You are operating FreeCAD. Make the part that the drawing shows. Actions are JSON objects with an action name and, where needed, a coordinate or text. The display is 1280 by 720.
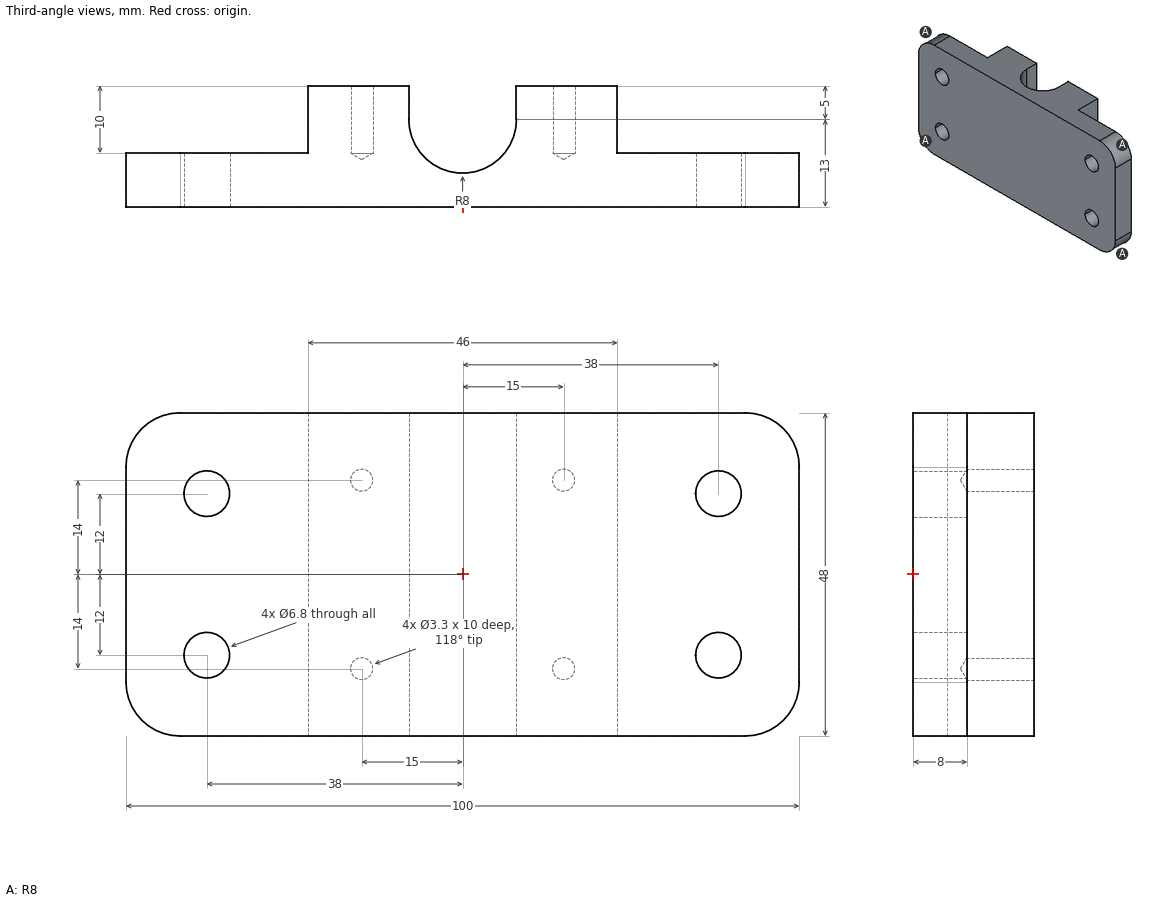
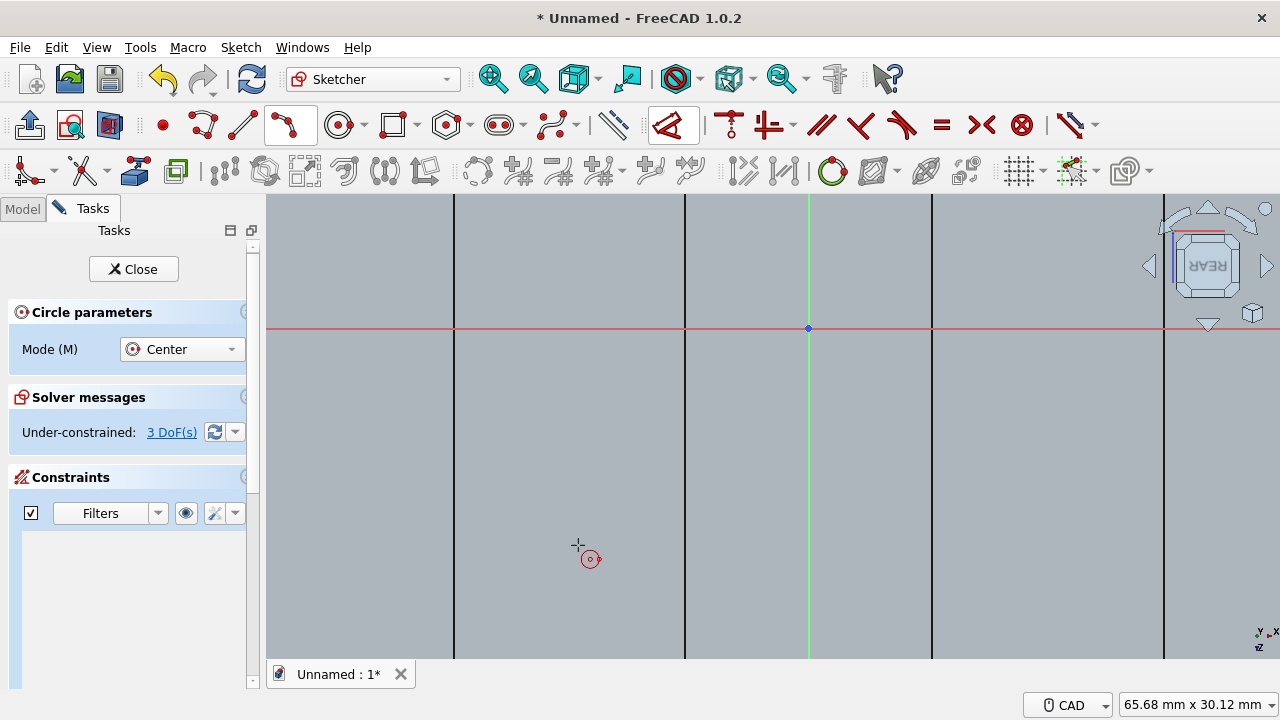
{"action": "left_click", "coordinate": [577, 545]}
{"action": "left_click", "coordinate": [595, 527]}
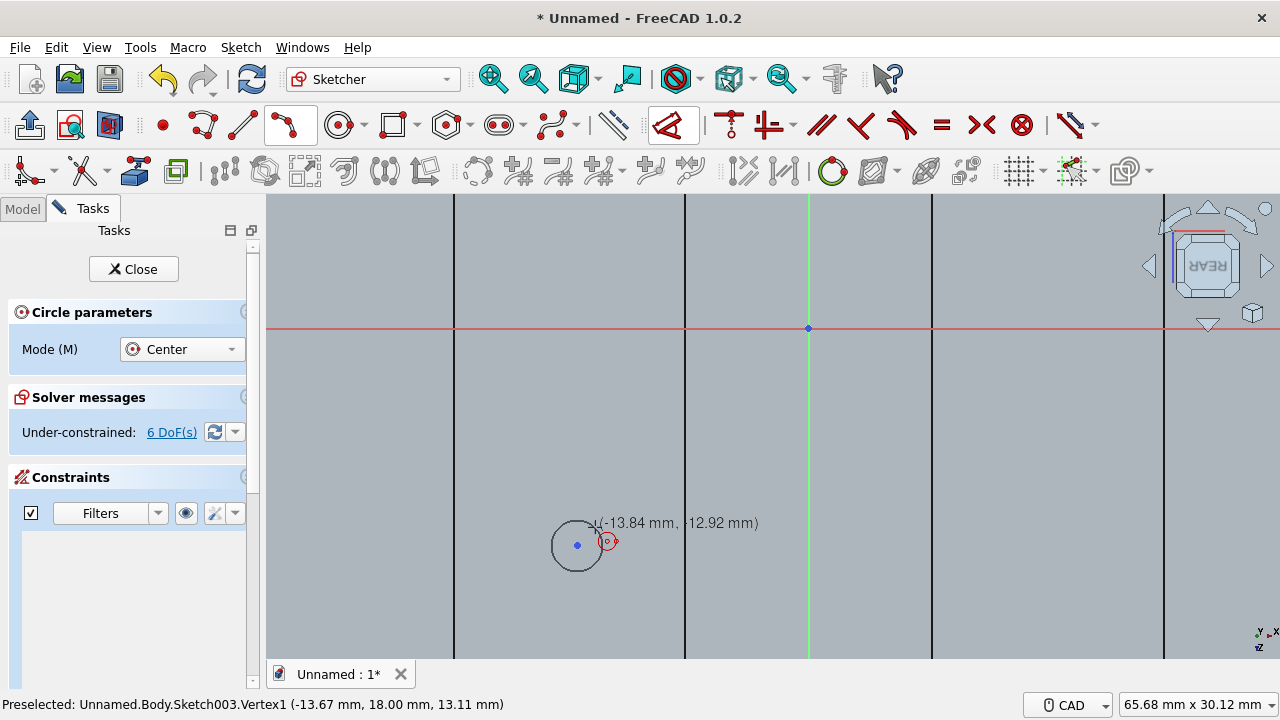
{"action": "left_click", "coordinate": [1040, 545]}
{"action": "left_click", "coordinate": [1058, 527]}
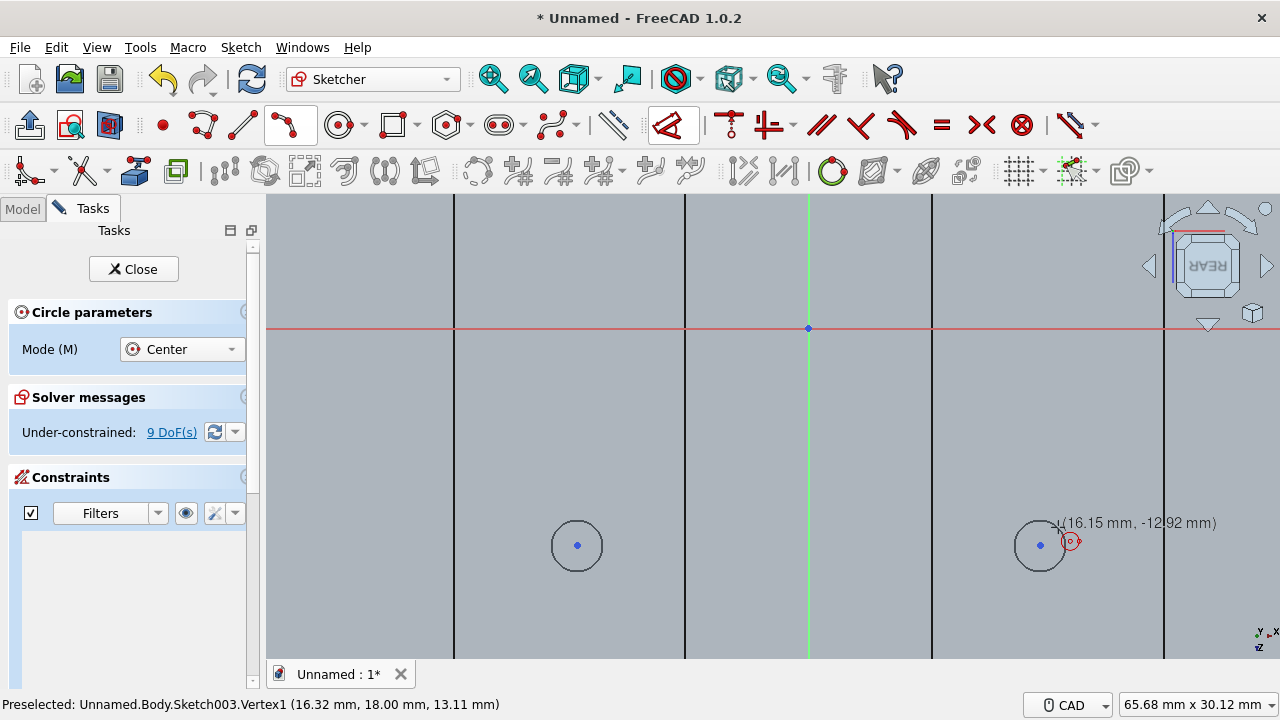
{"action": "scroll", "coordinate": [578, 546], "scroll_direction": "down", "scroll_amount": 3}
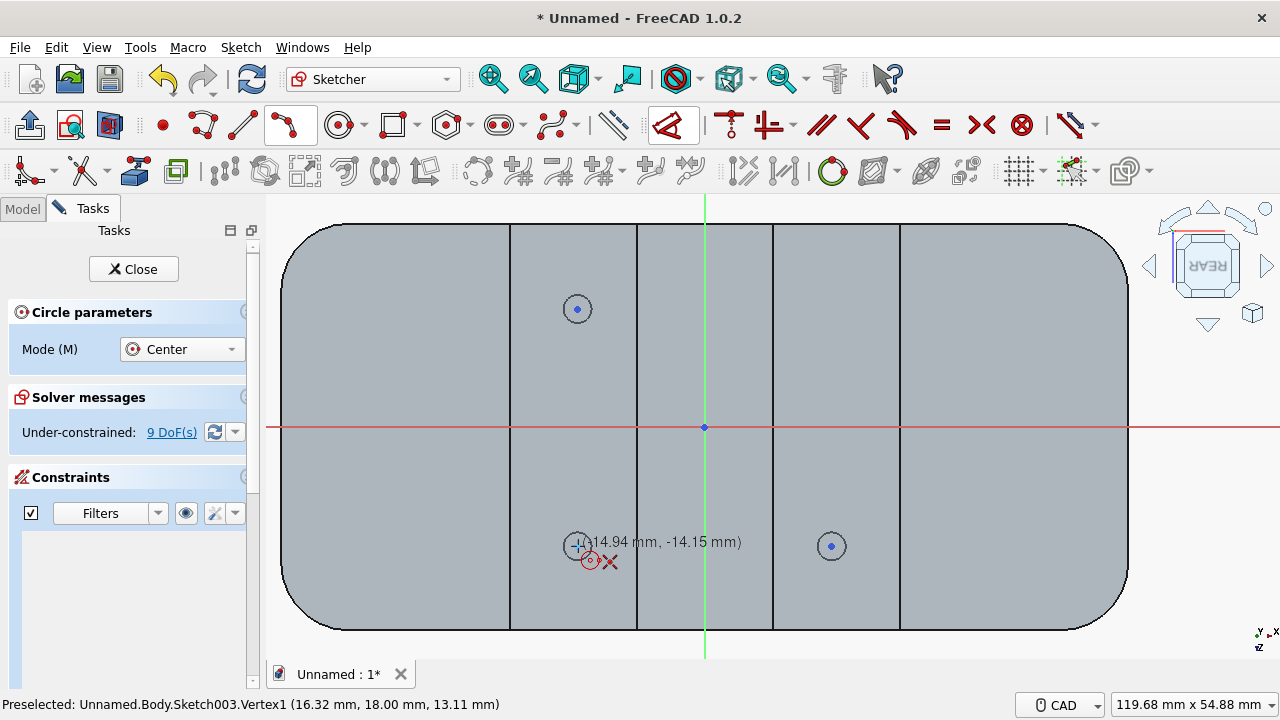
{"action": "scroll", "coordinate": [832, 308], "scroll_direction": "up", "scroll_amount": 3}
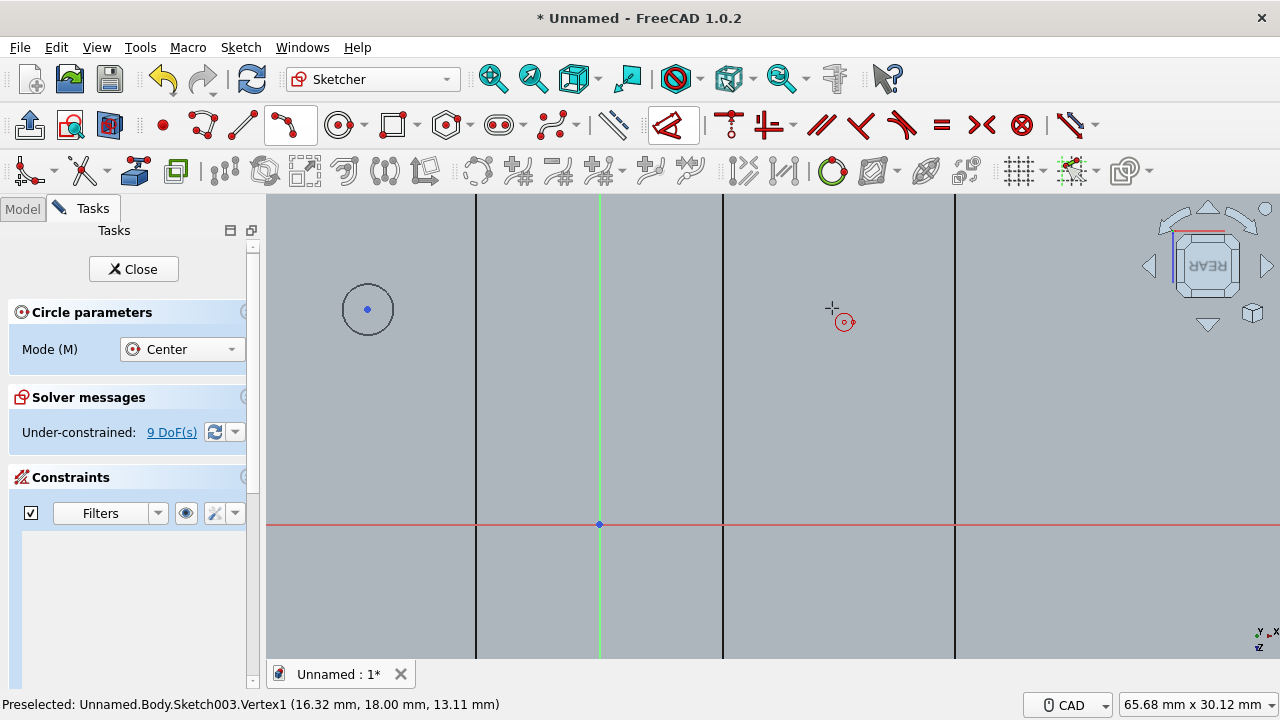
{"action": "left_click", "coordinate": [831, 309]}
{"action": "left_click", "coordinate": [849, 291]}
{"action": "key", "text": "Escape"}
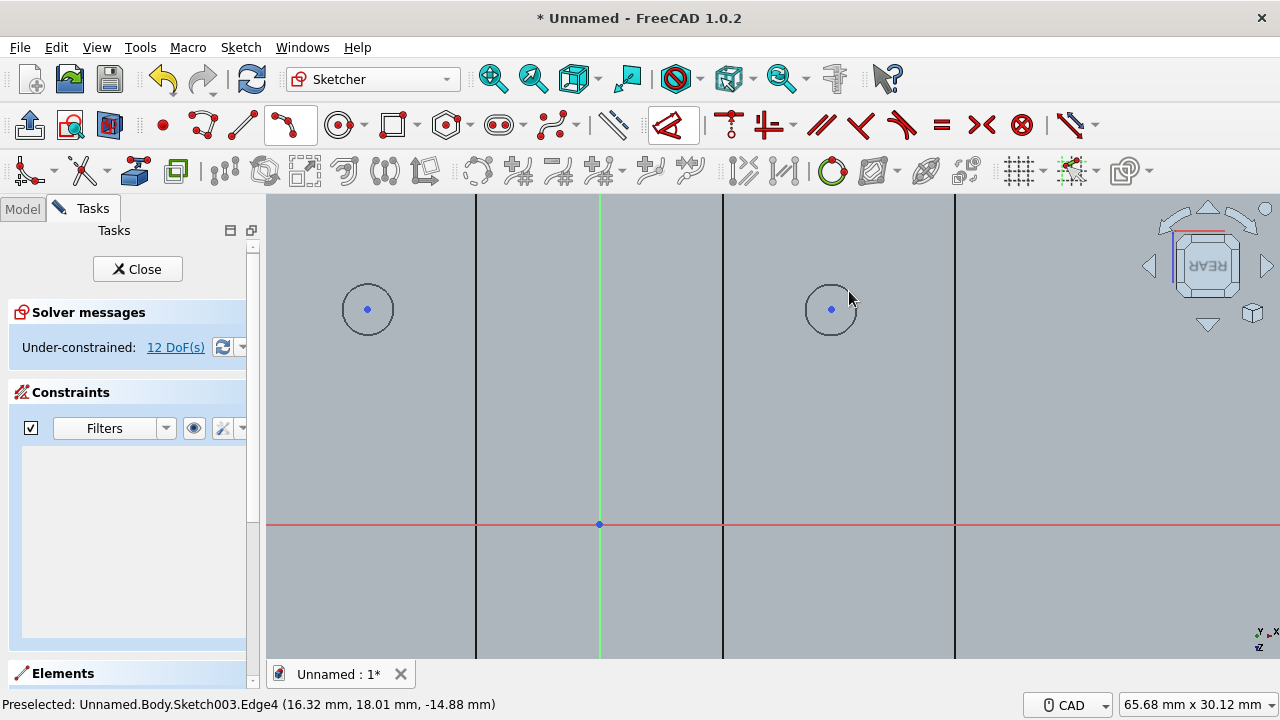
{"action": "left_click", "coordinate": [386, 292]}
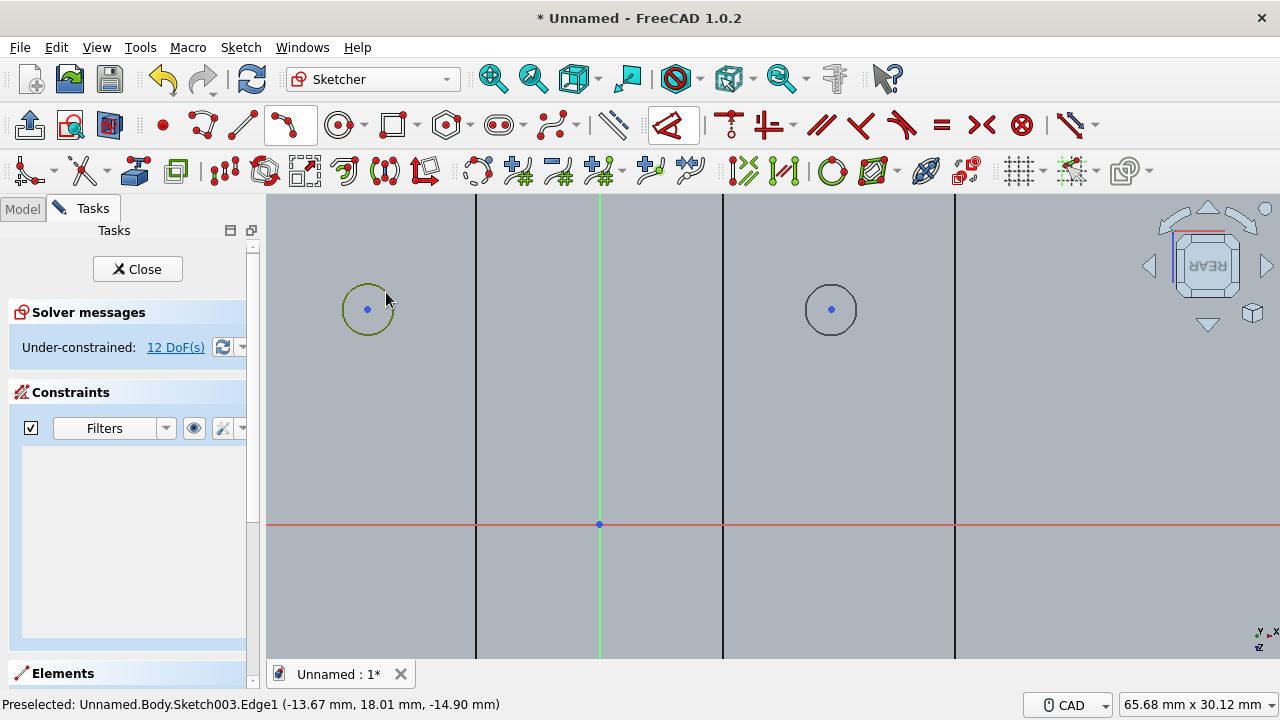
{"action": "scroll", "coordinate": [832, 307], "scroll_direction": "down", "scroll_amount": 3}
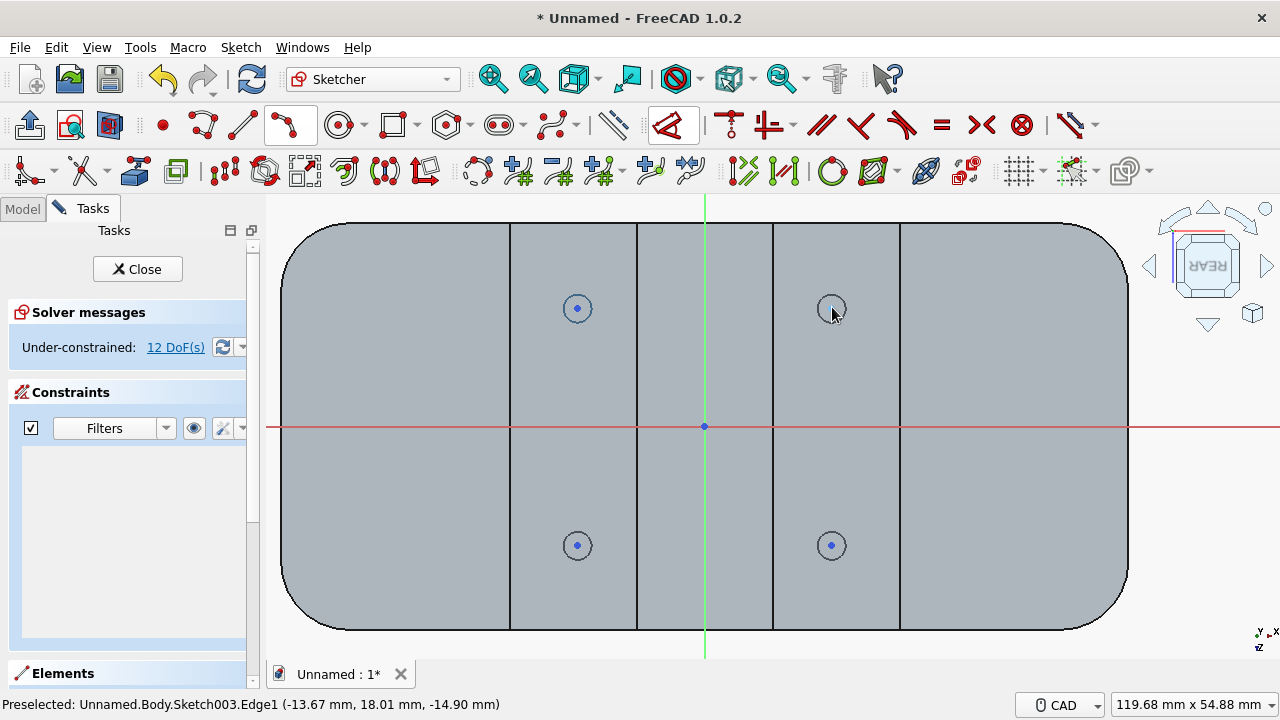
{"action": "left_click", "coordinate": [587, 536]}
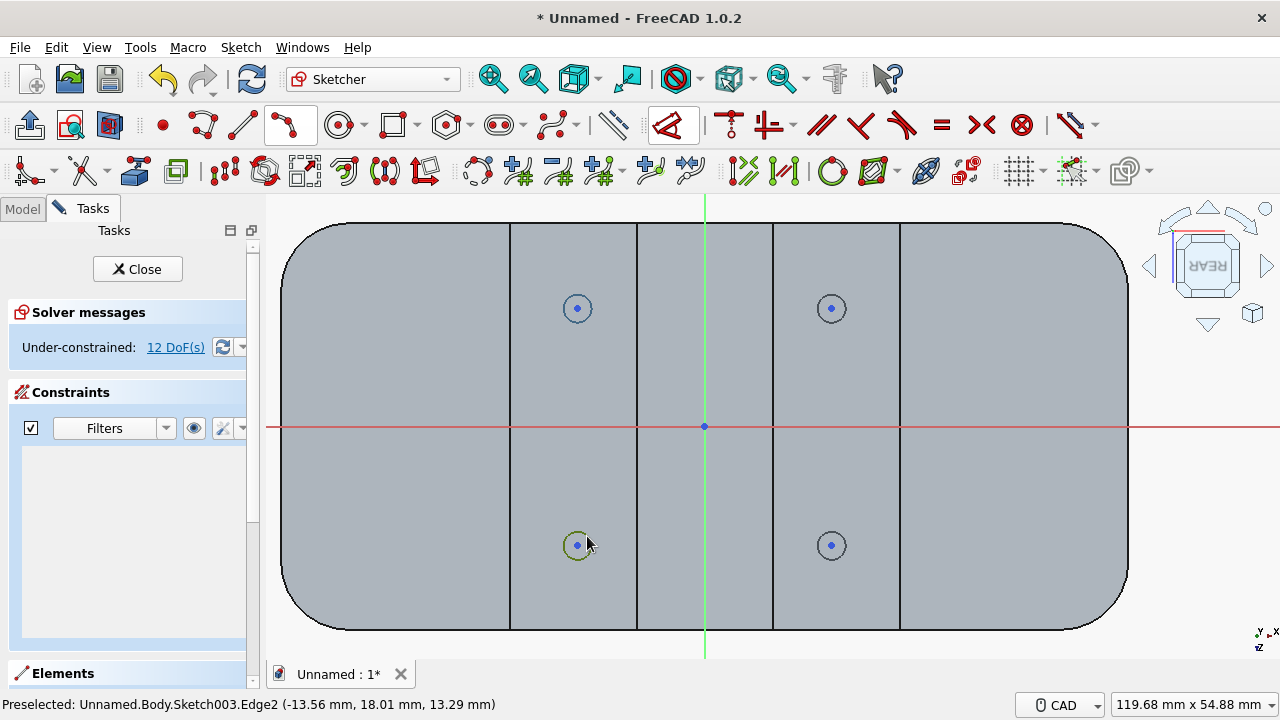
{"action": "left_click", "coordinate": [842, 536]}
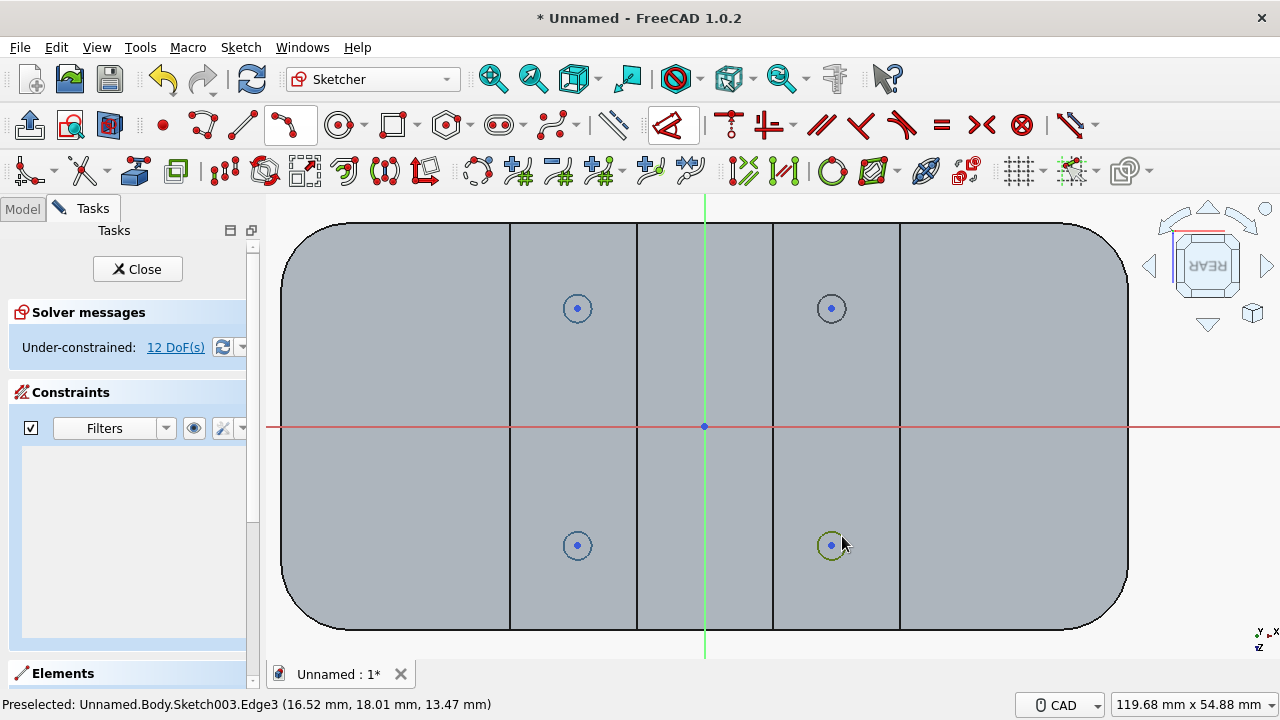
{"action": "left_click", "coordinate": [842, 299]}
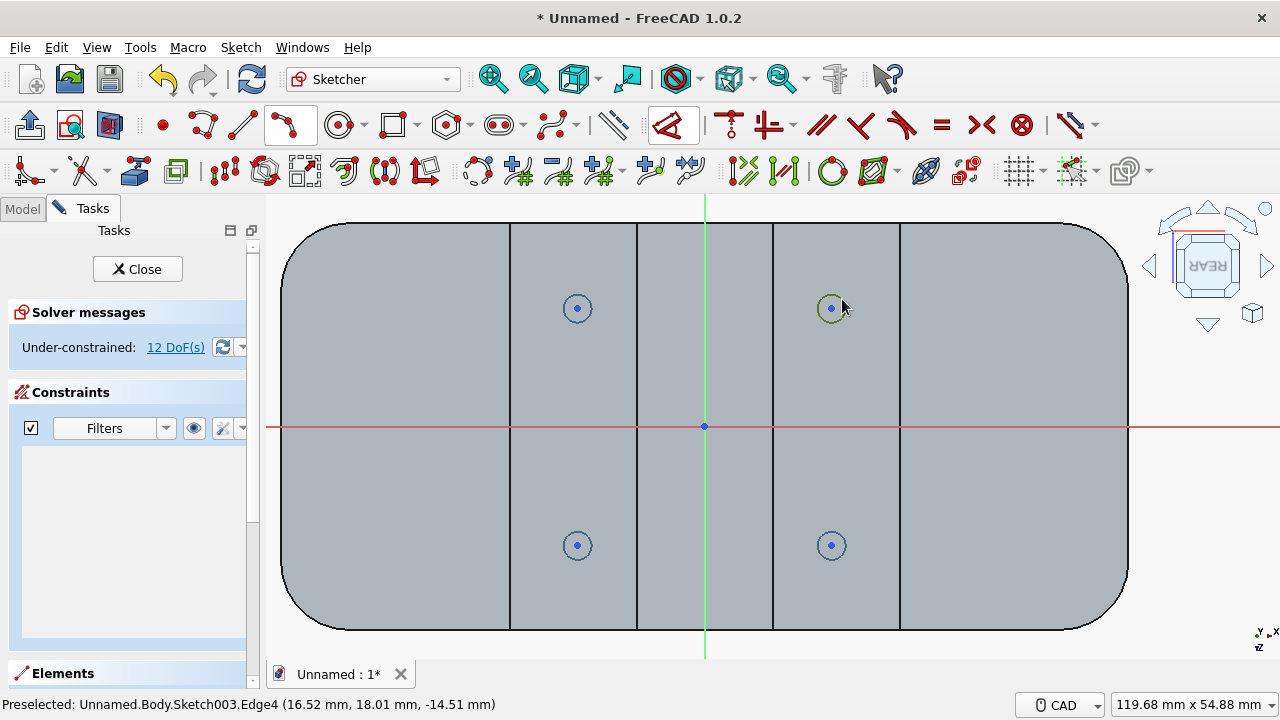
{"action": "left_click", "coordinate": [942, 126]}